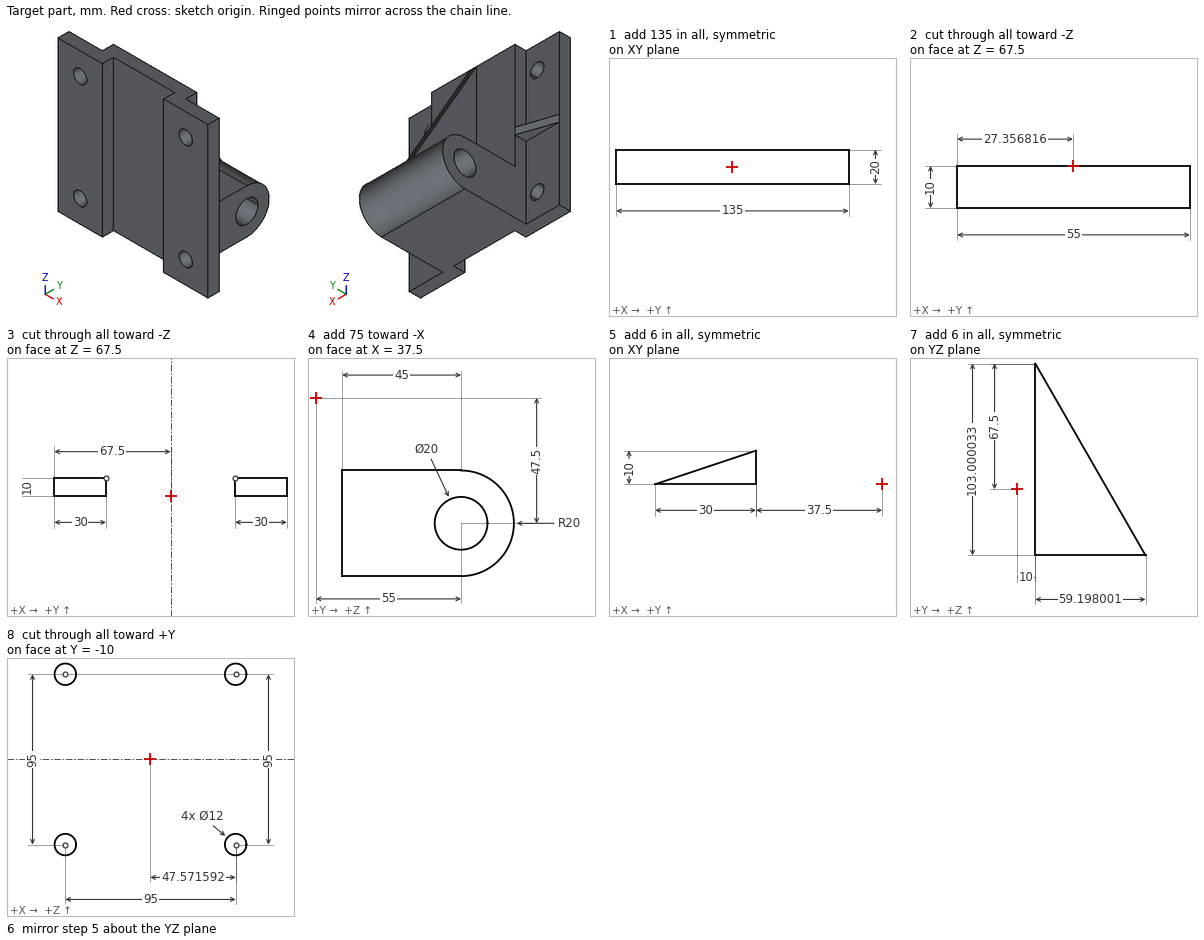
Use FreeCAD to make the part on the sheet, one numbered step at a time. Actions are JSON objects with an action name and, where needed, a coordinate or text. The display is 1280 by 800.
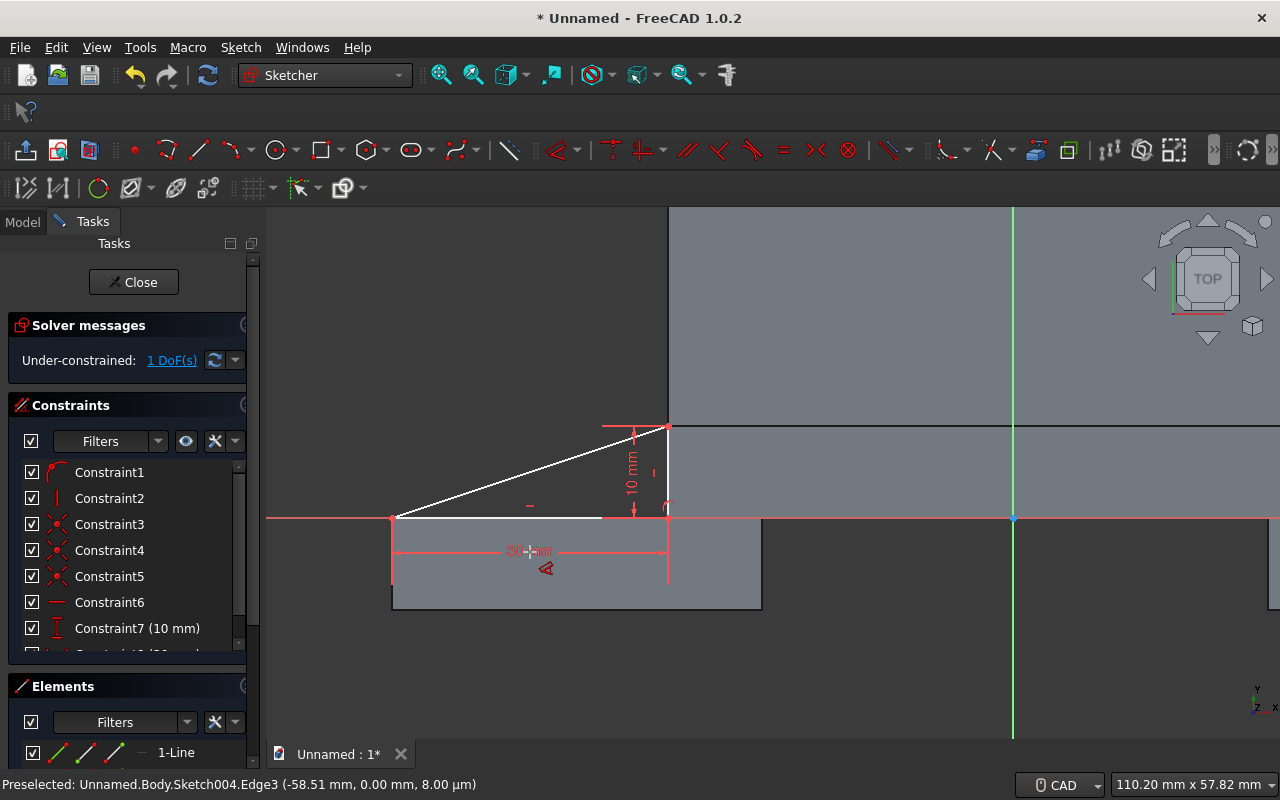
{"action": "left_click", "coordinate": [668, 518]}
{"action": "left_click", "coordinate": [841, 552]}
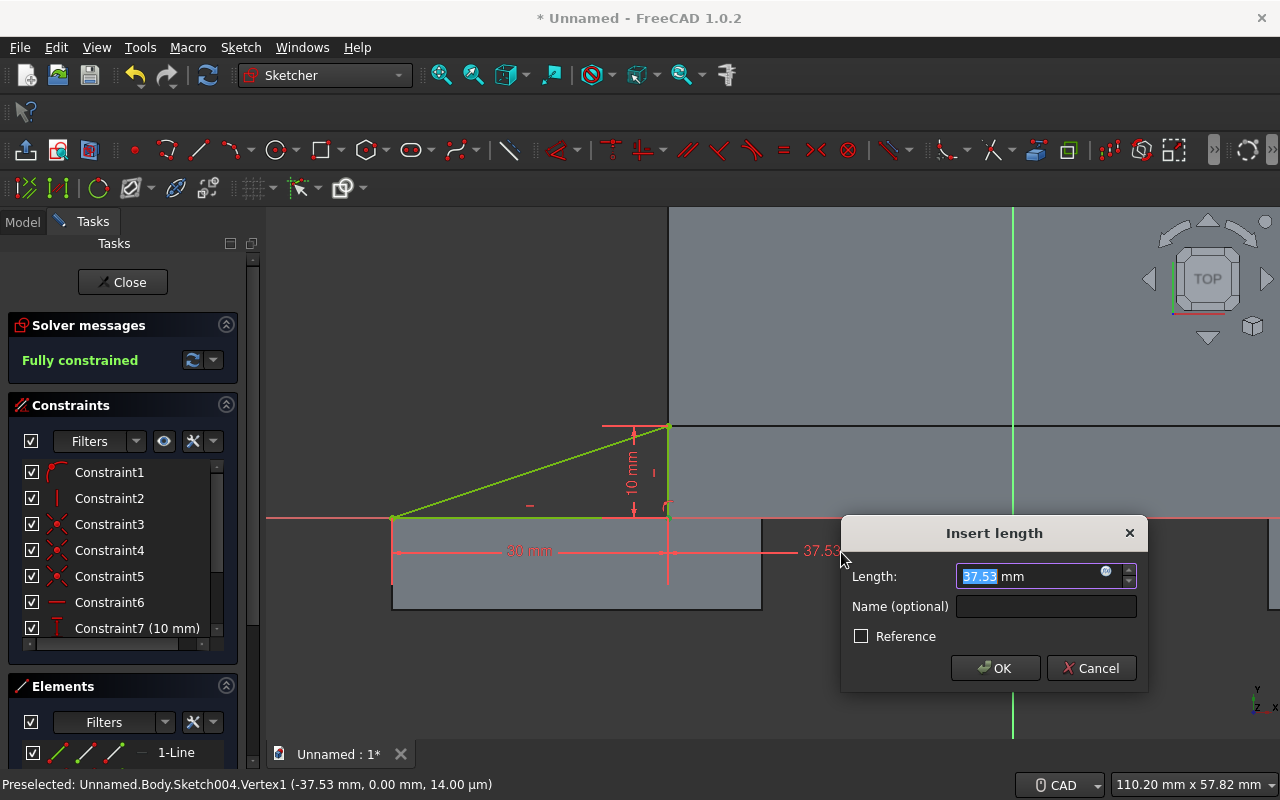
{"action": "type", "text": "37.5"}
{"action": "key", "text": "Return"}
{"action": "key", "text": "Escape"}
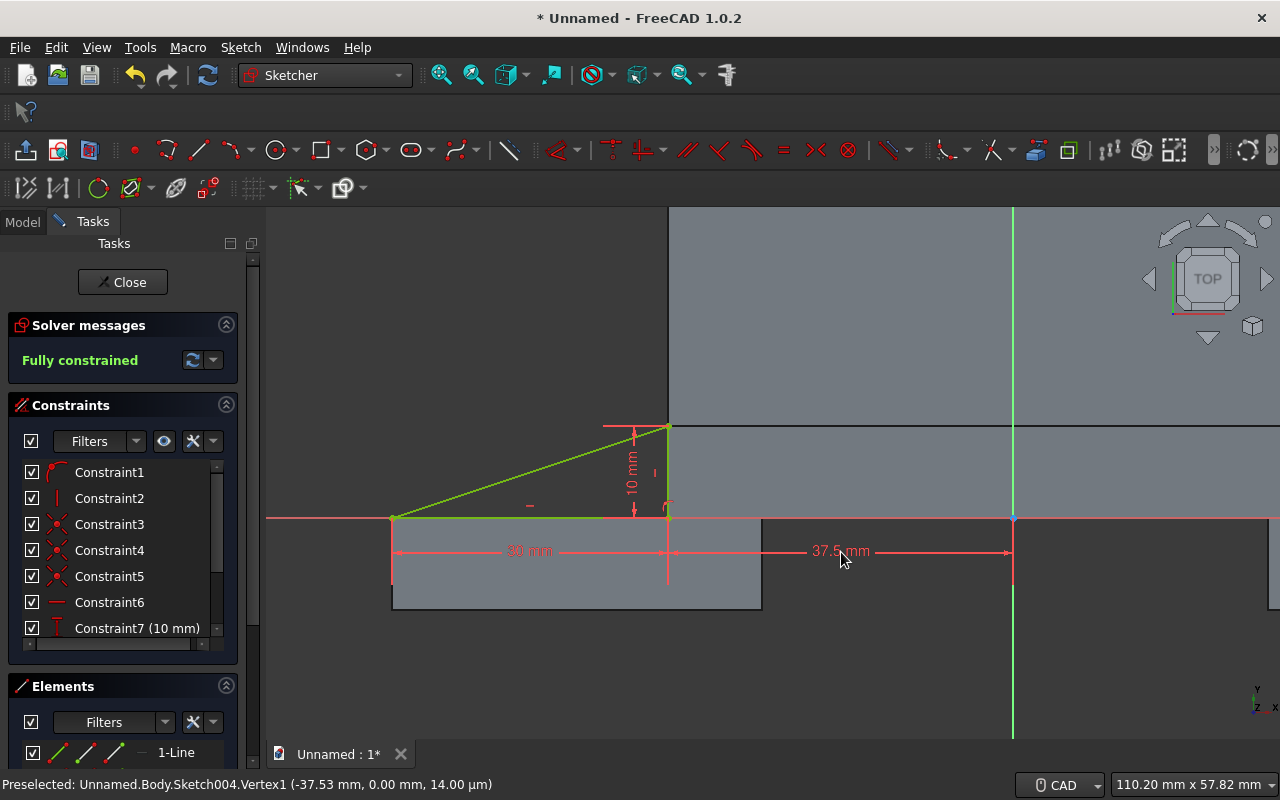
{"action": "left_click", "coordinate": [123, 282]}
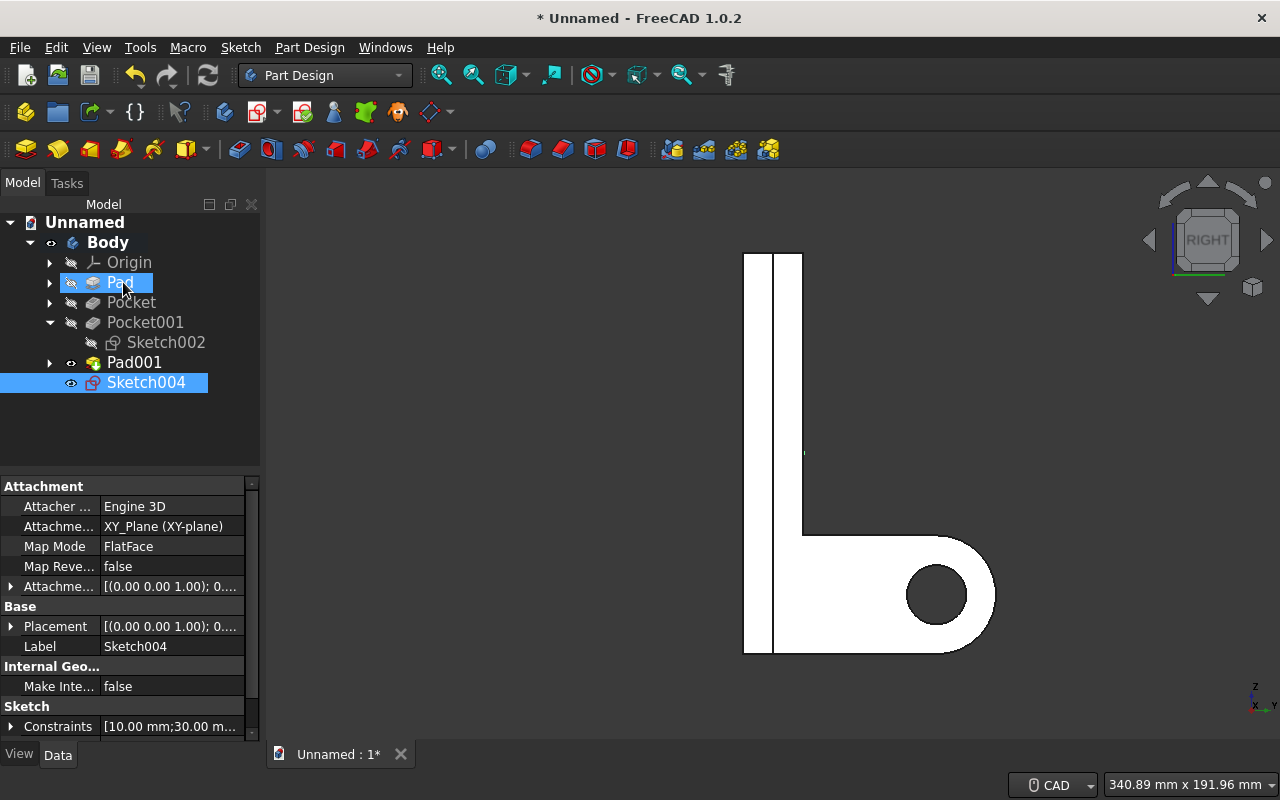
{"action": "left_click", "coordinate": [26, 150]}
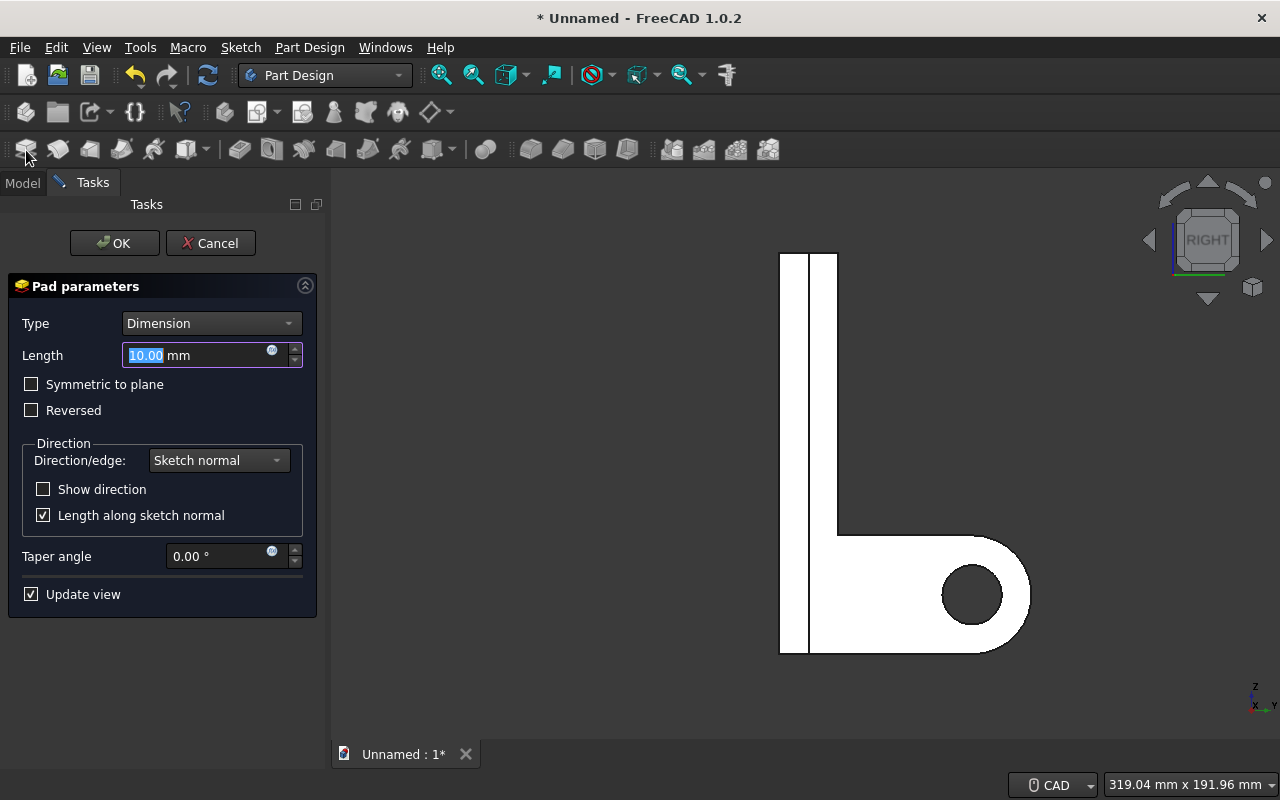
{"action": "type", "text": "6"}
{"action": "key", "text": "Tab"}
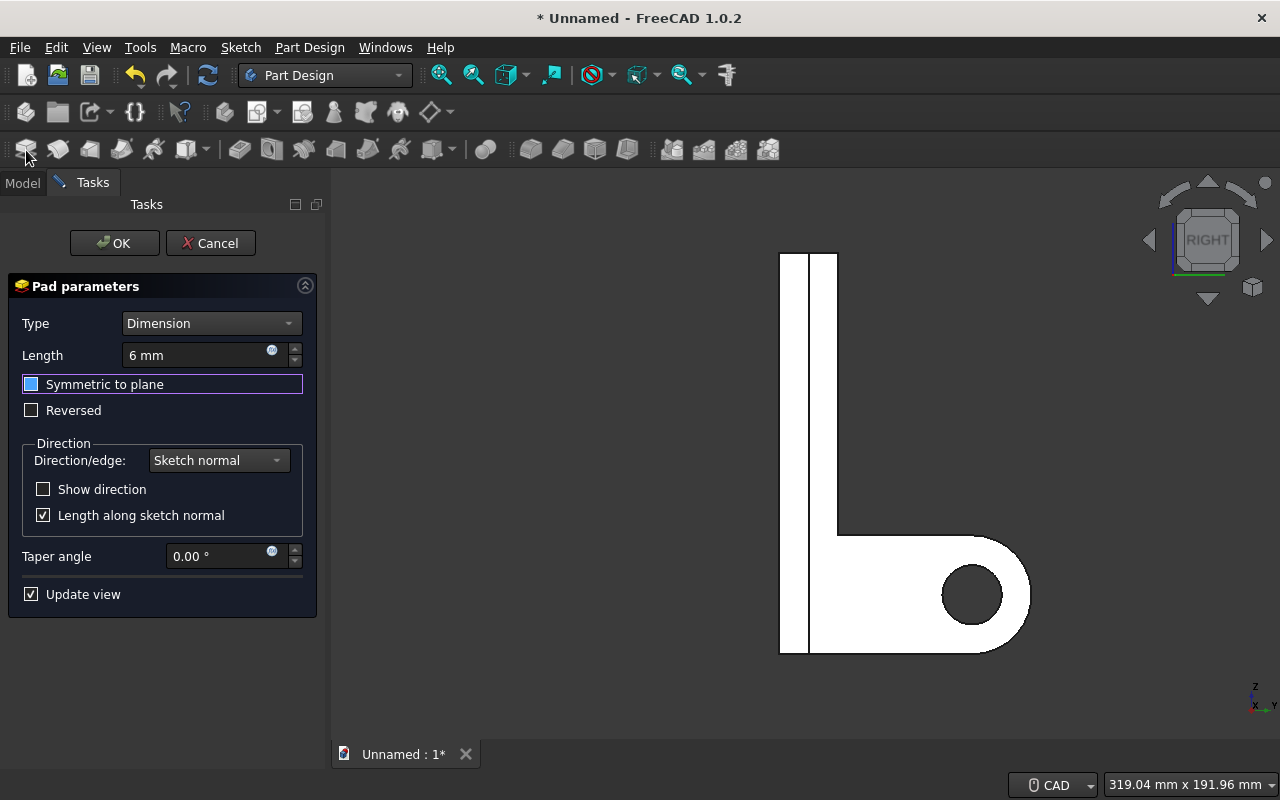
{"action": "left_click", "coordinate": [30, 384]}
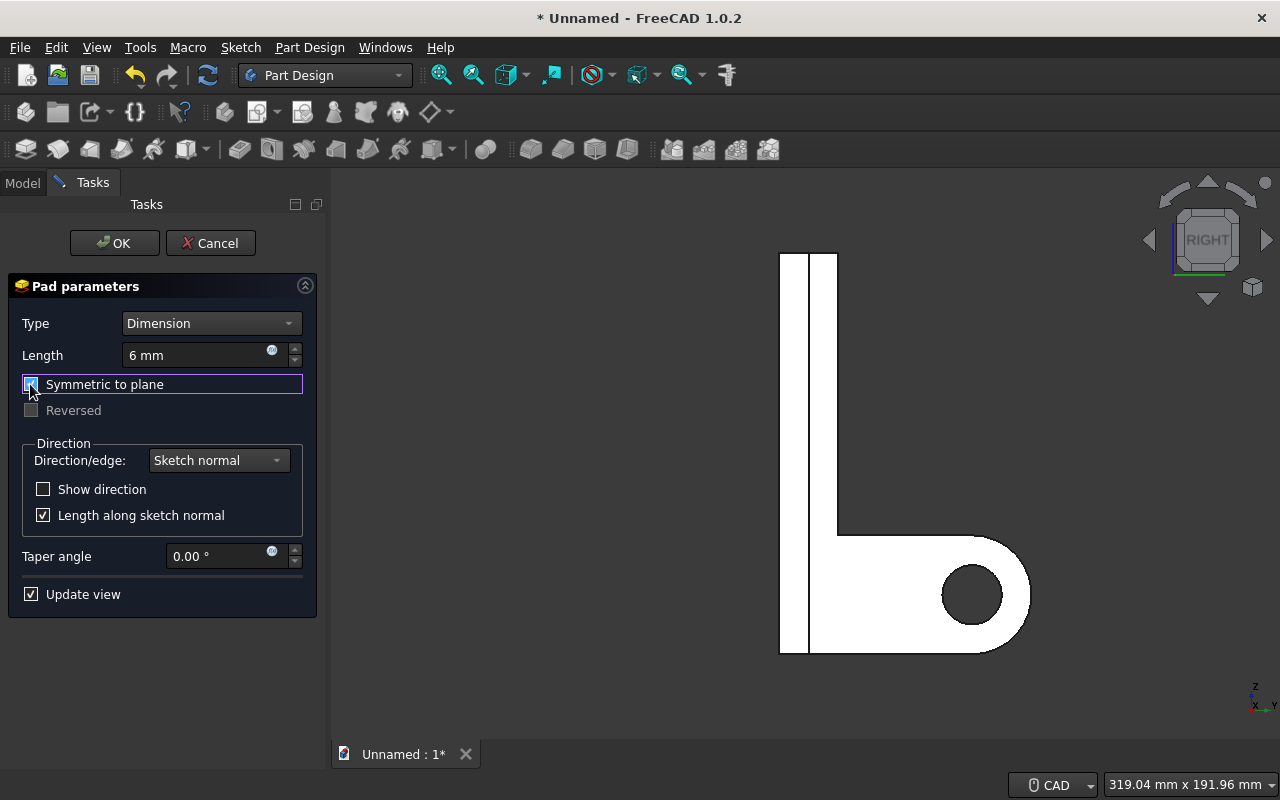
{"action": "left_click", "coordinate": [115, 243]}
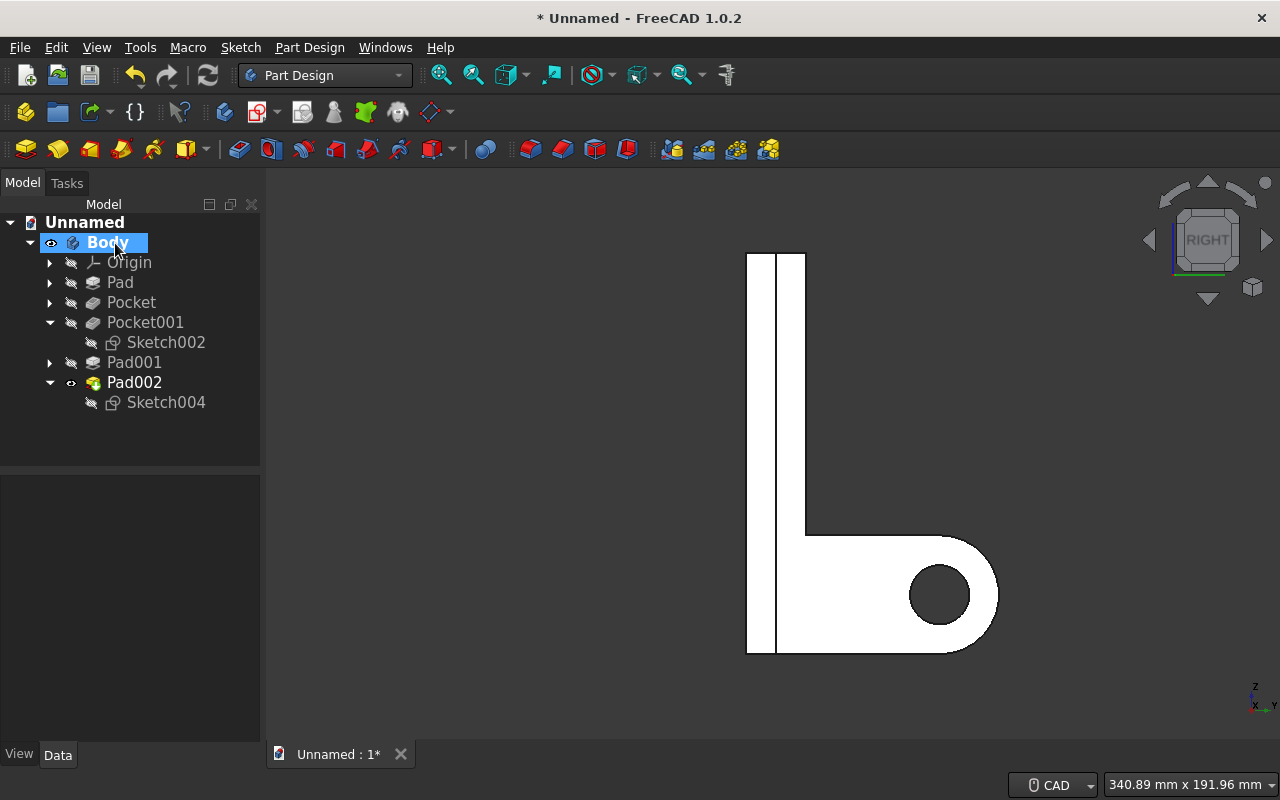
{"action": "left_click", "coordinate": [116, 383]}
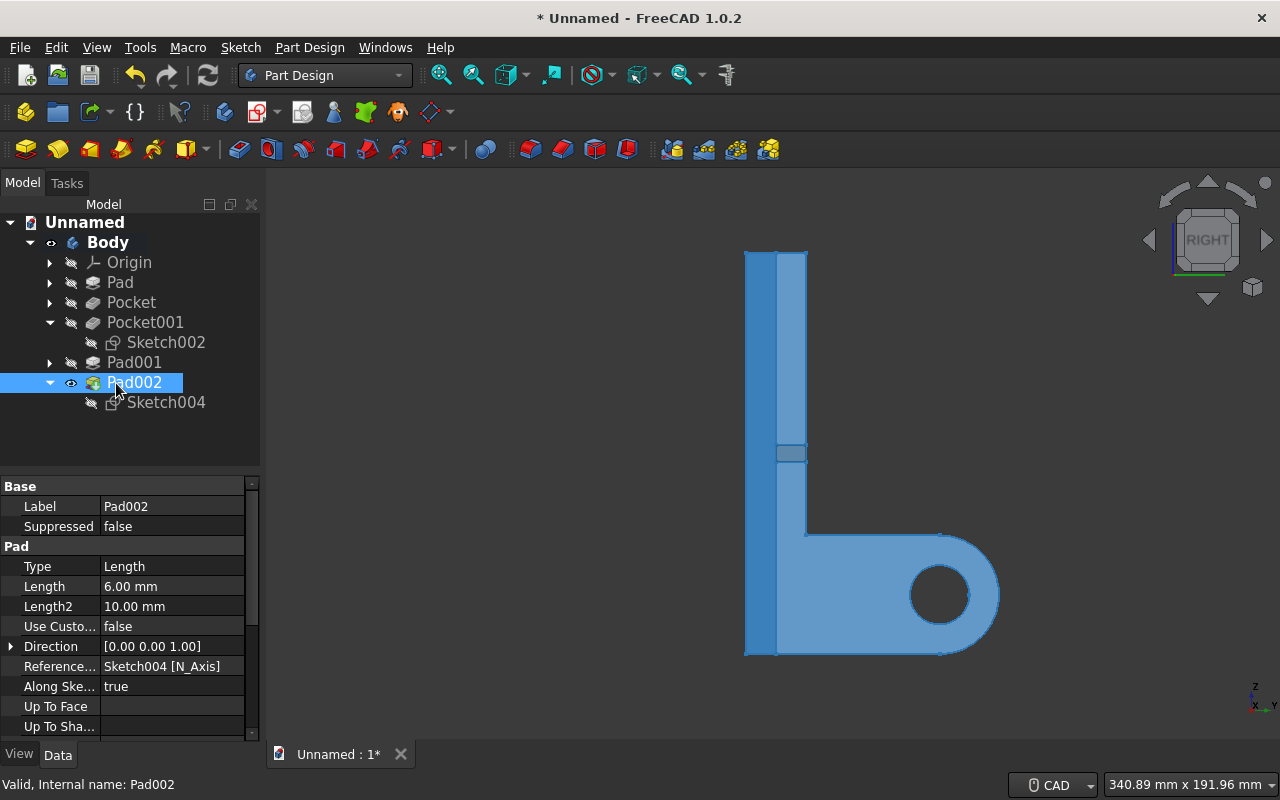
{"action": "left_click", "coordinate": [672, 150]}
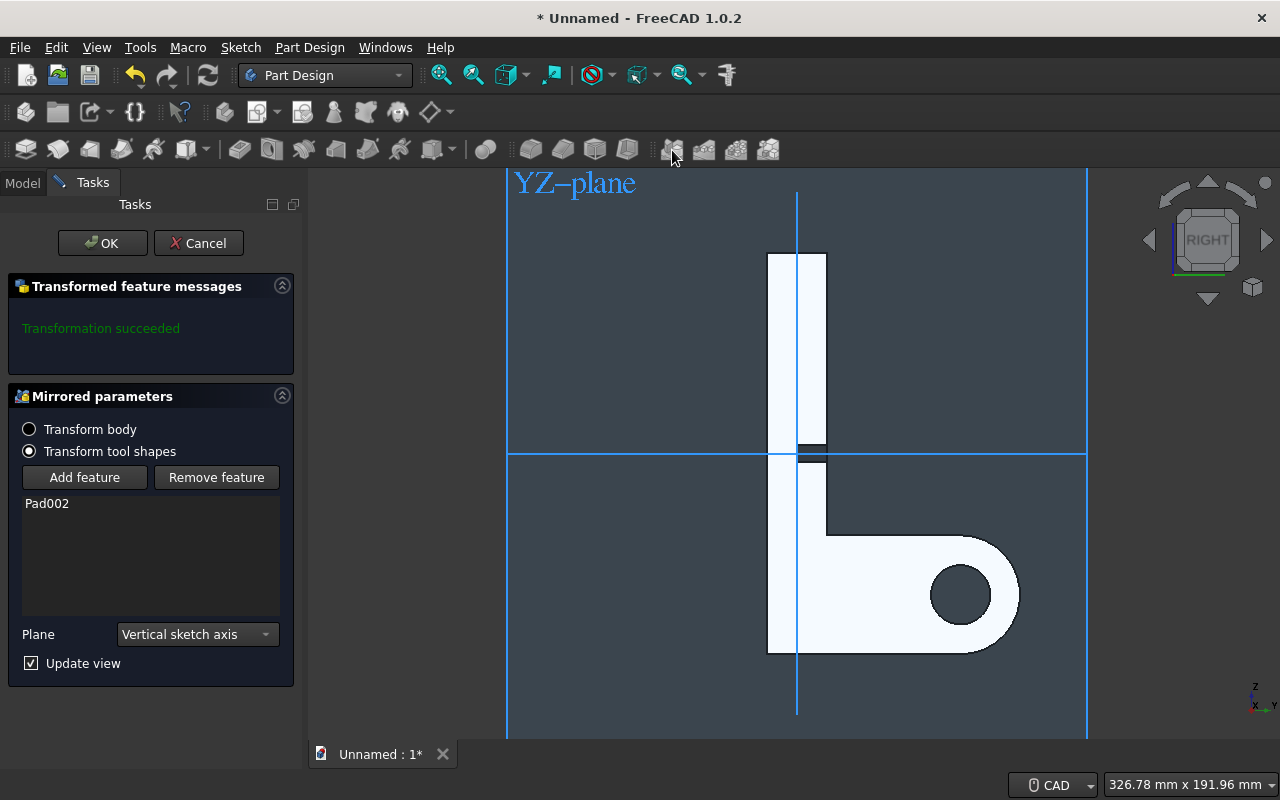
{"action": "left_click", "coordinate": [198, 634]}